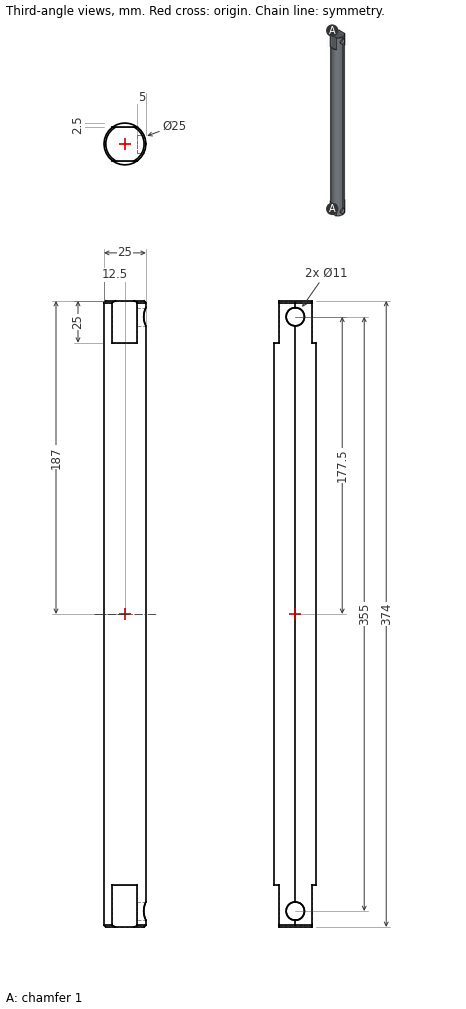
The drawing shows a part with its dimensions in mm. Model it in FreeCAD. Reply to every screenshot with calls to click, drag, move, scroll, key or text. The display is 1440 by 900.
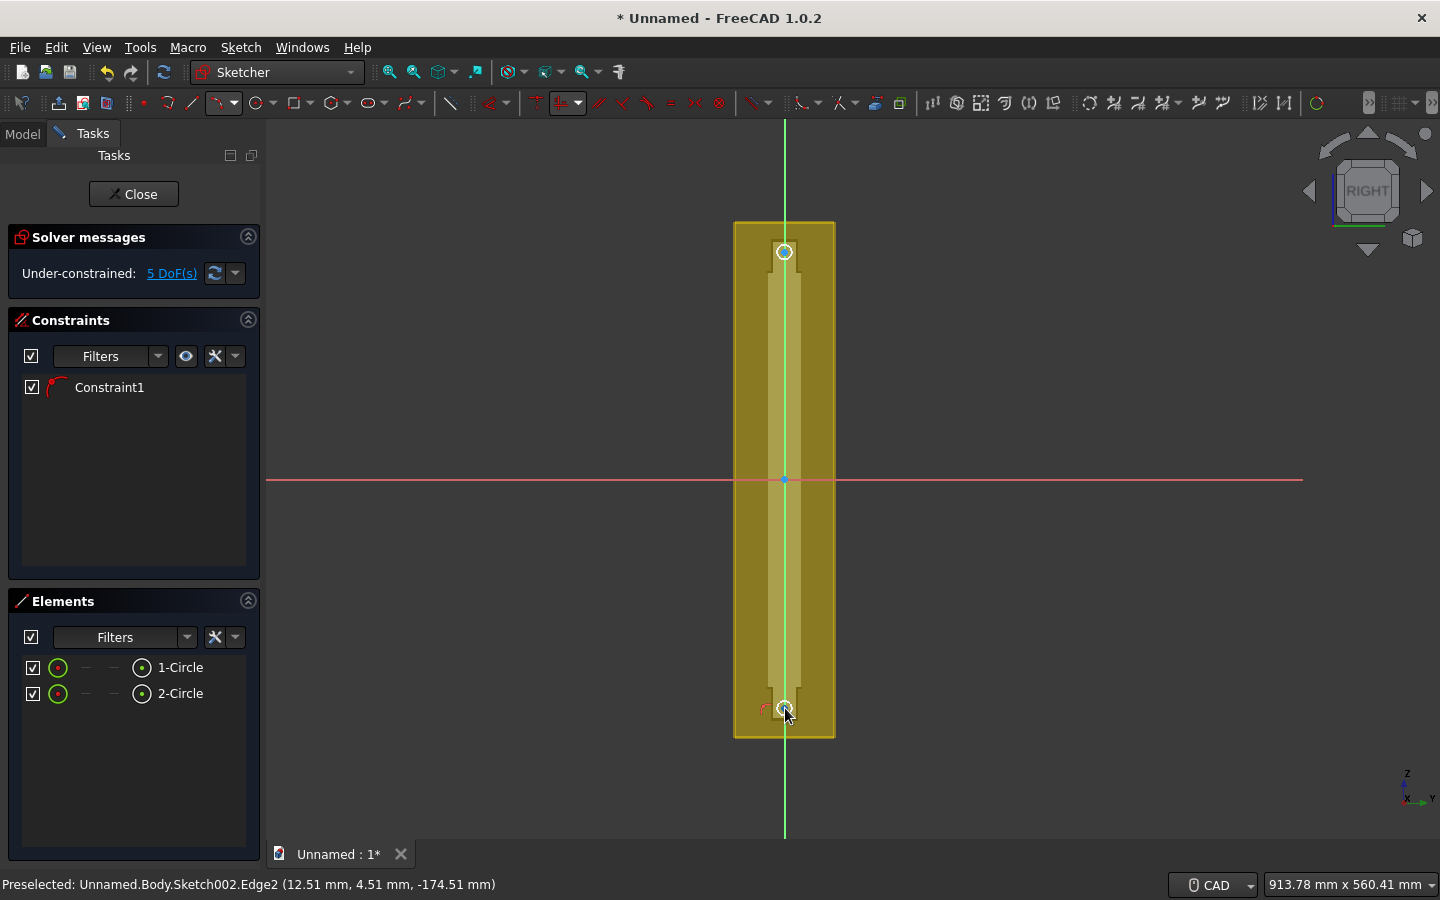
scroll(790, 247, up, 6)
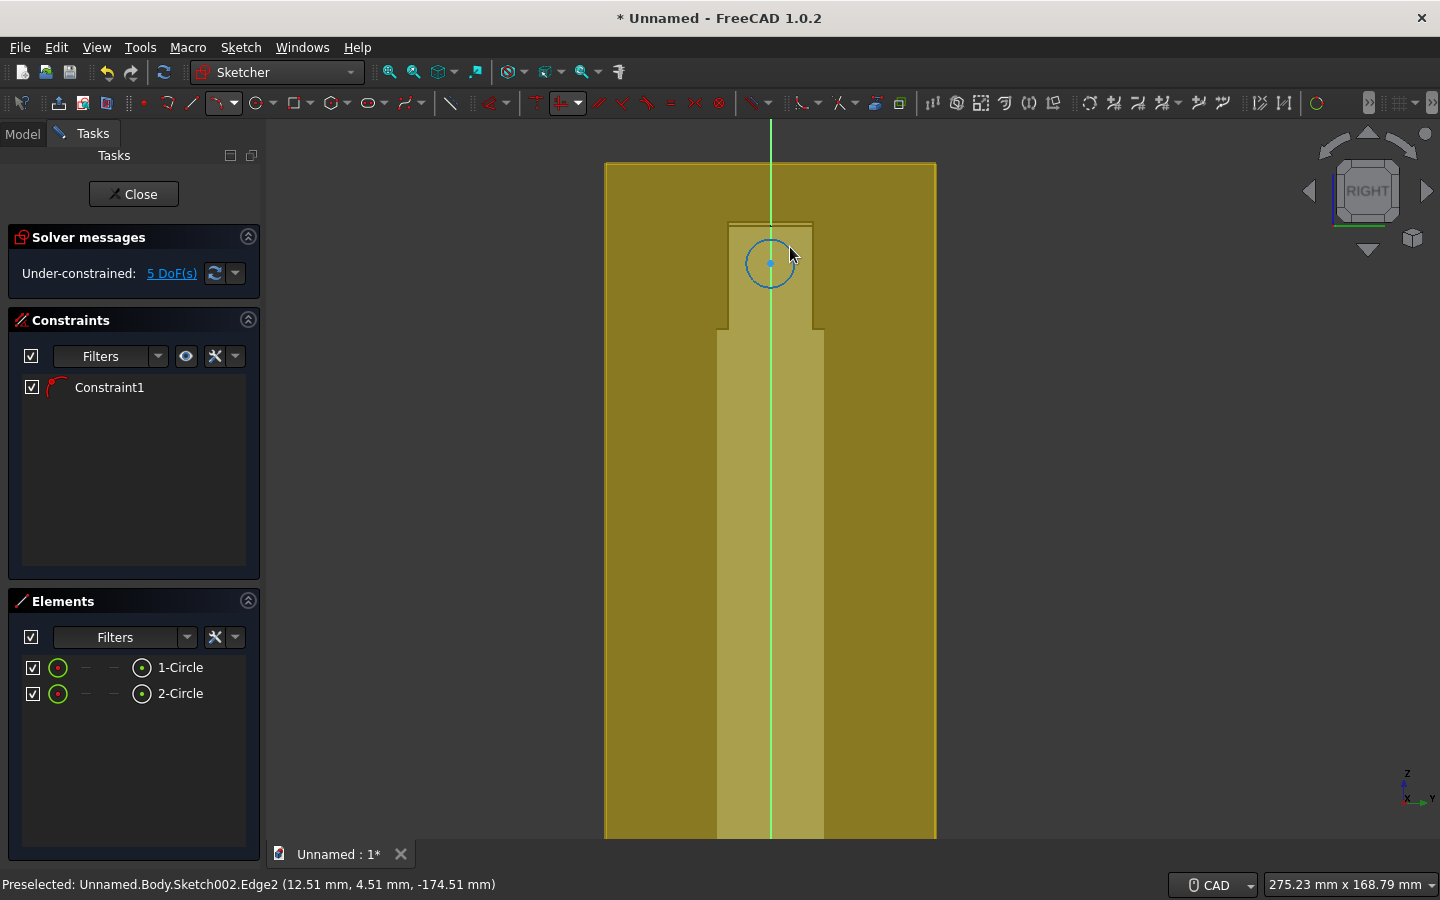
click(787, 247)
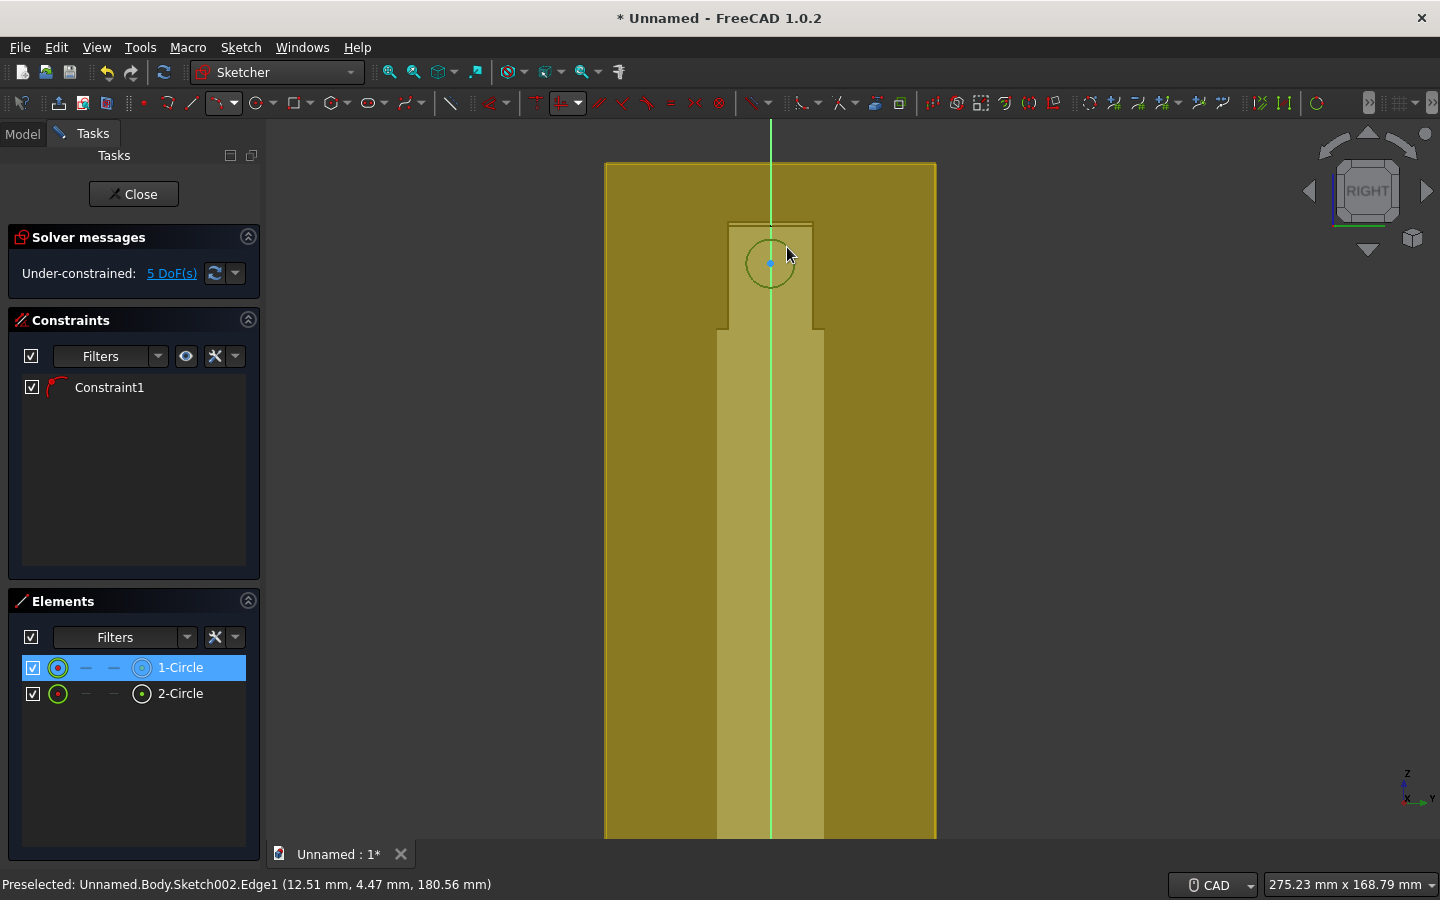
scroll(790, 246, down, 6)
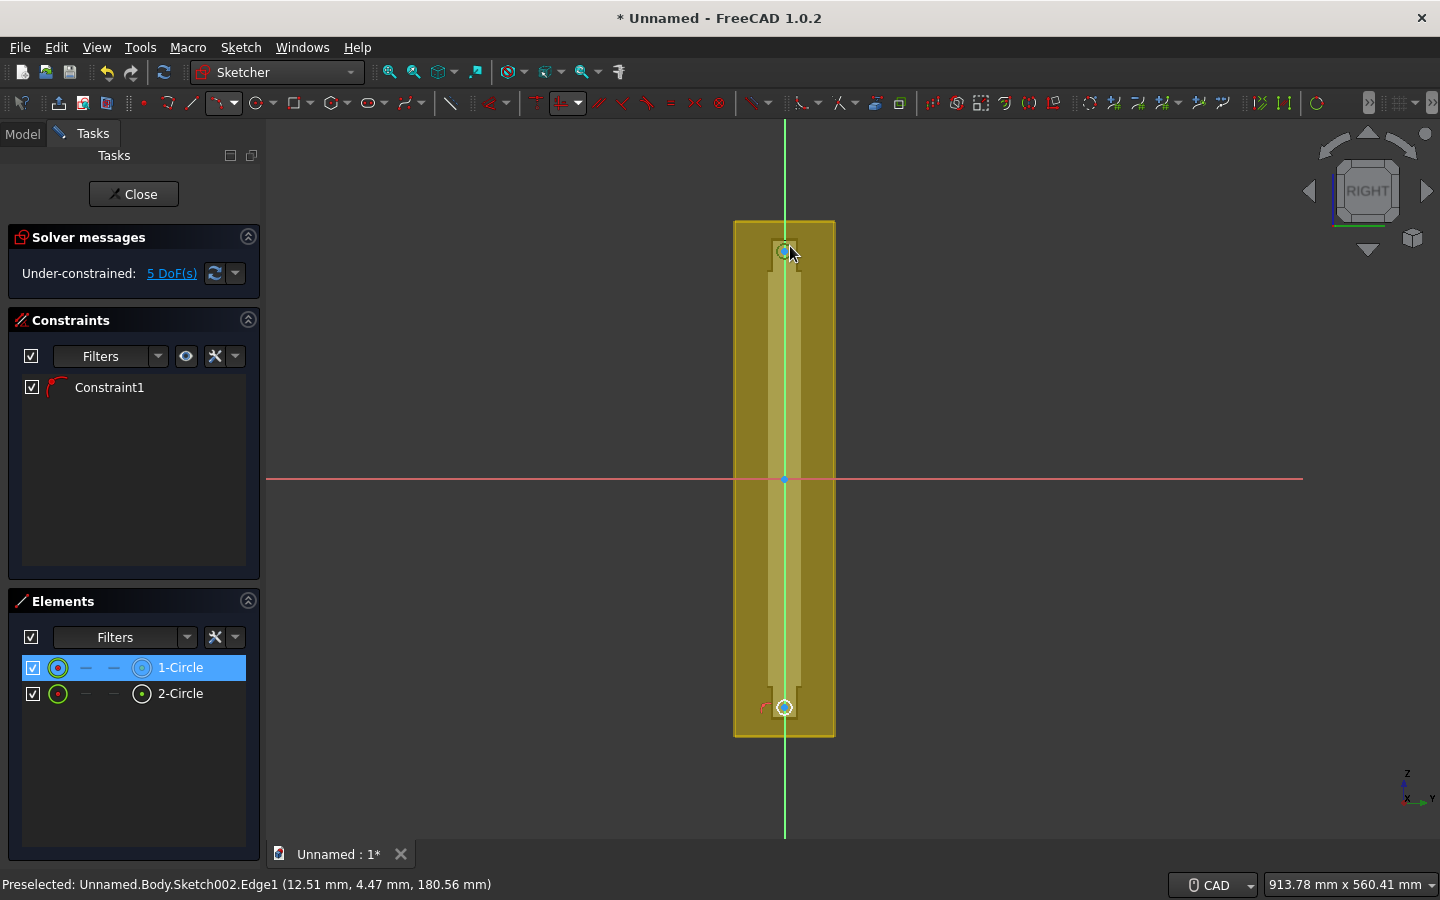
scroll(790, 702, up, 6)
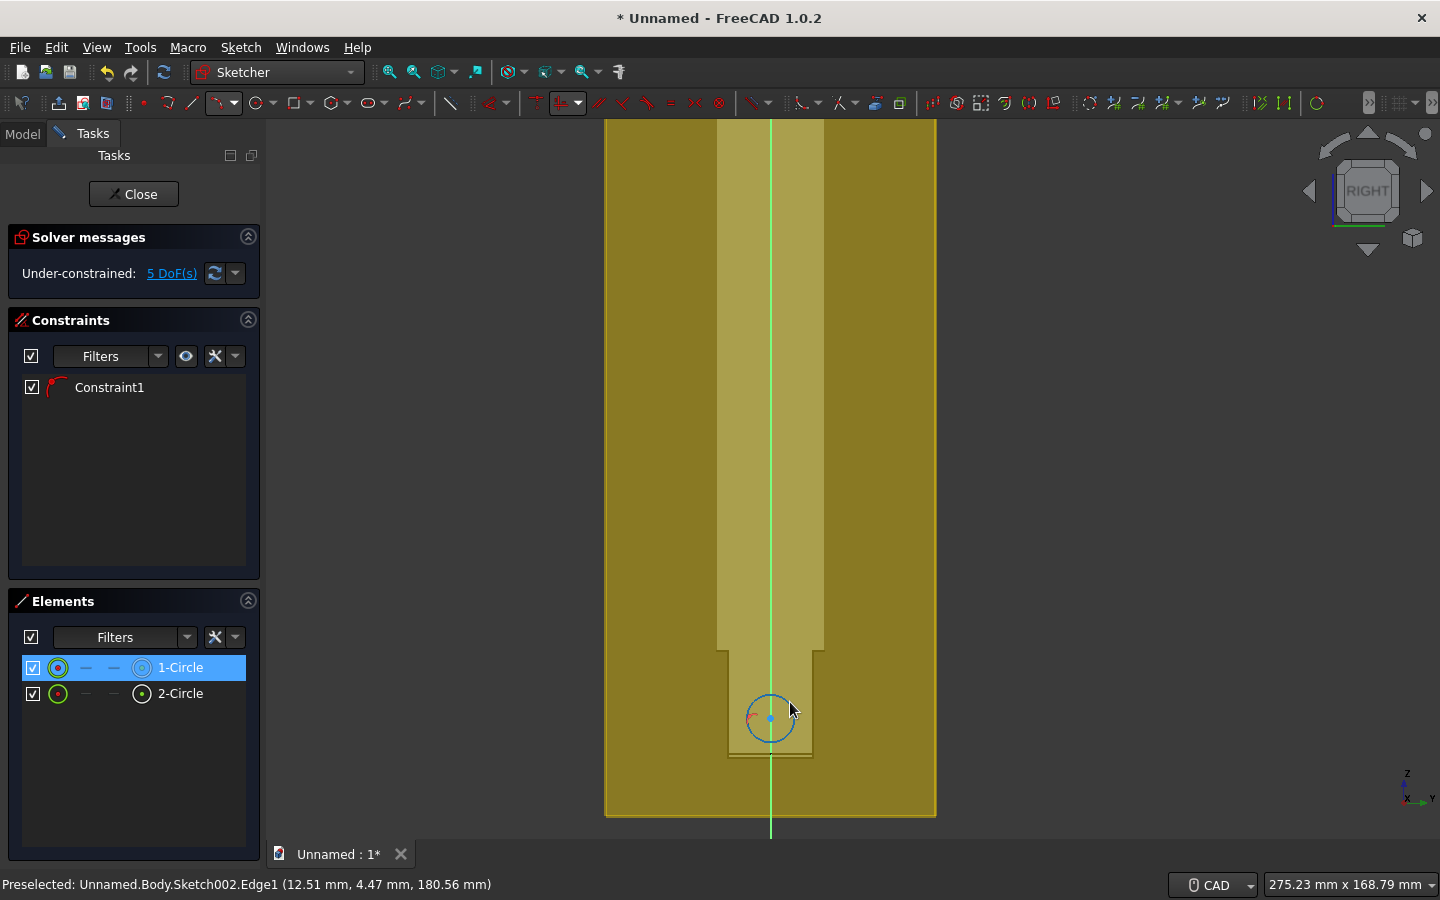
click(788, 702)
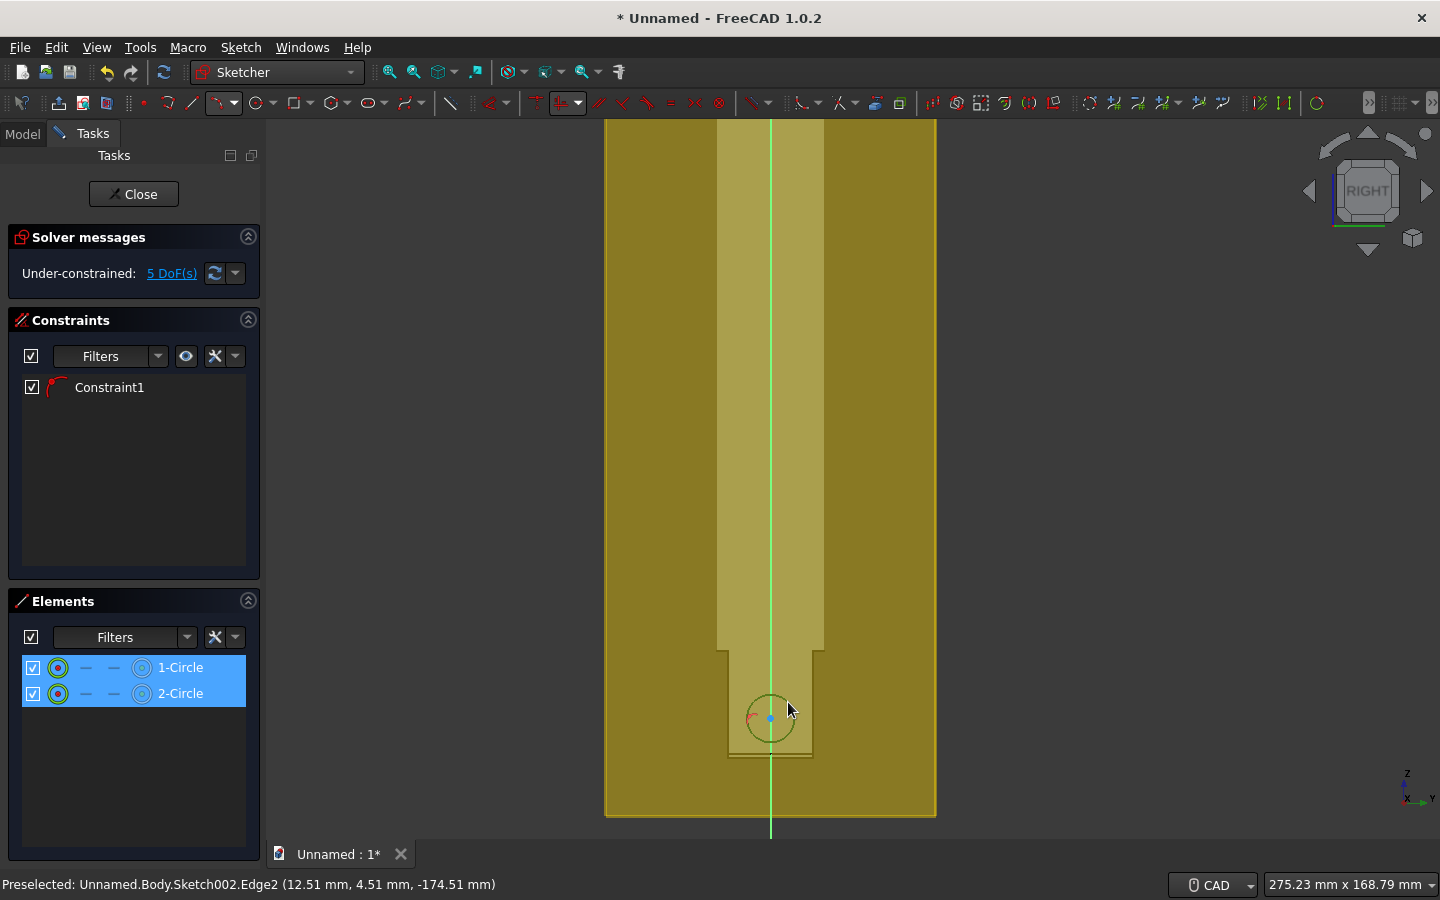
click(672, 104)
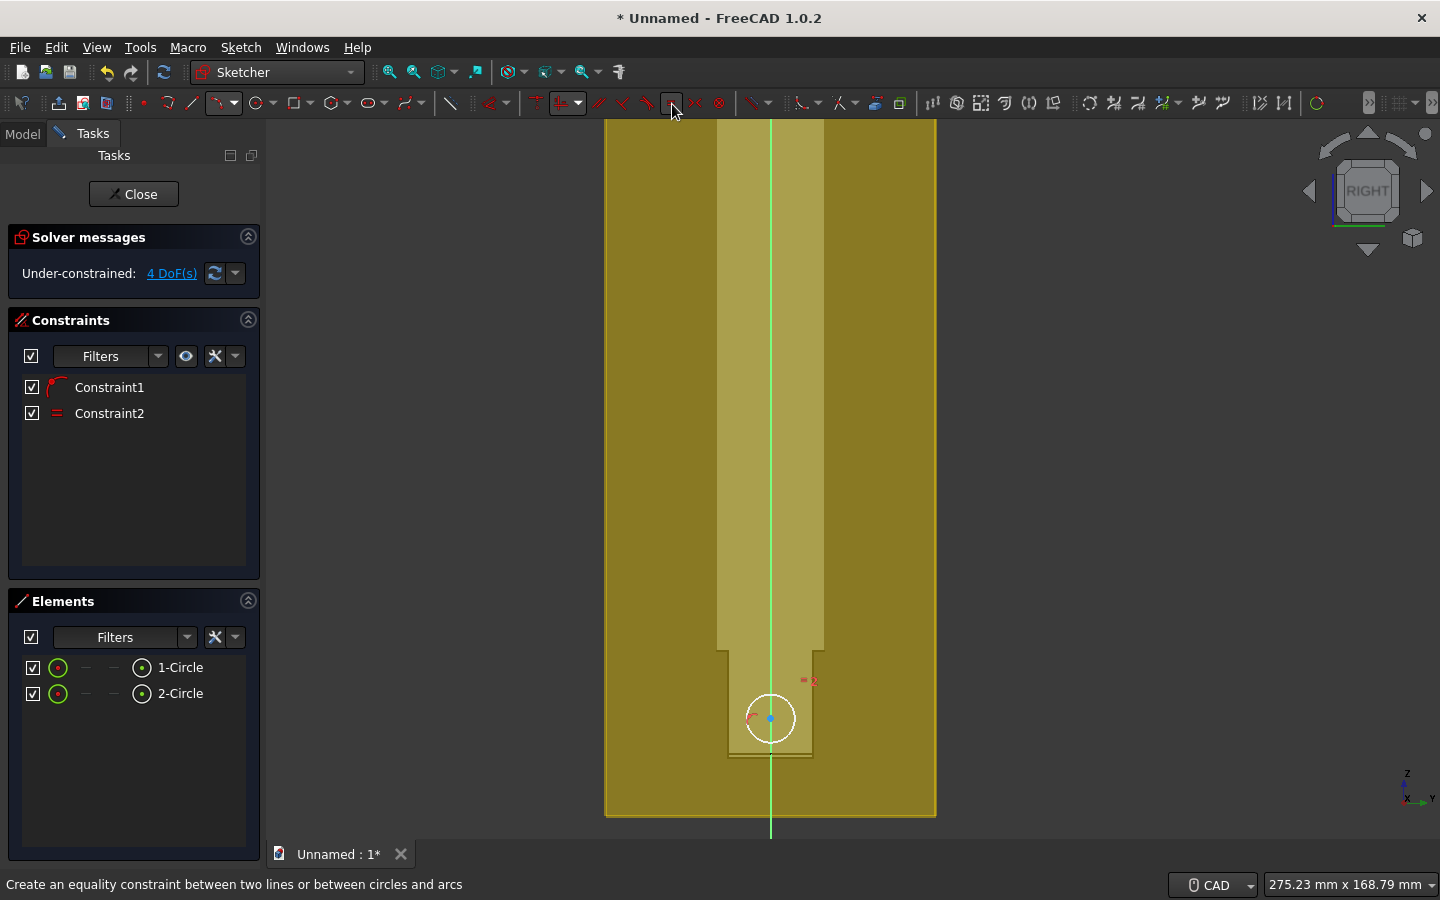
scroll(790, 703, down, 6)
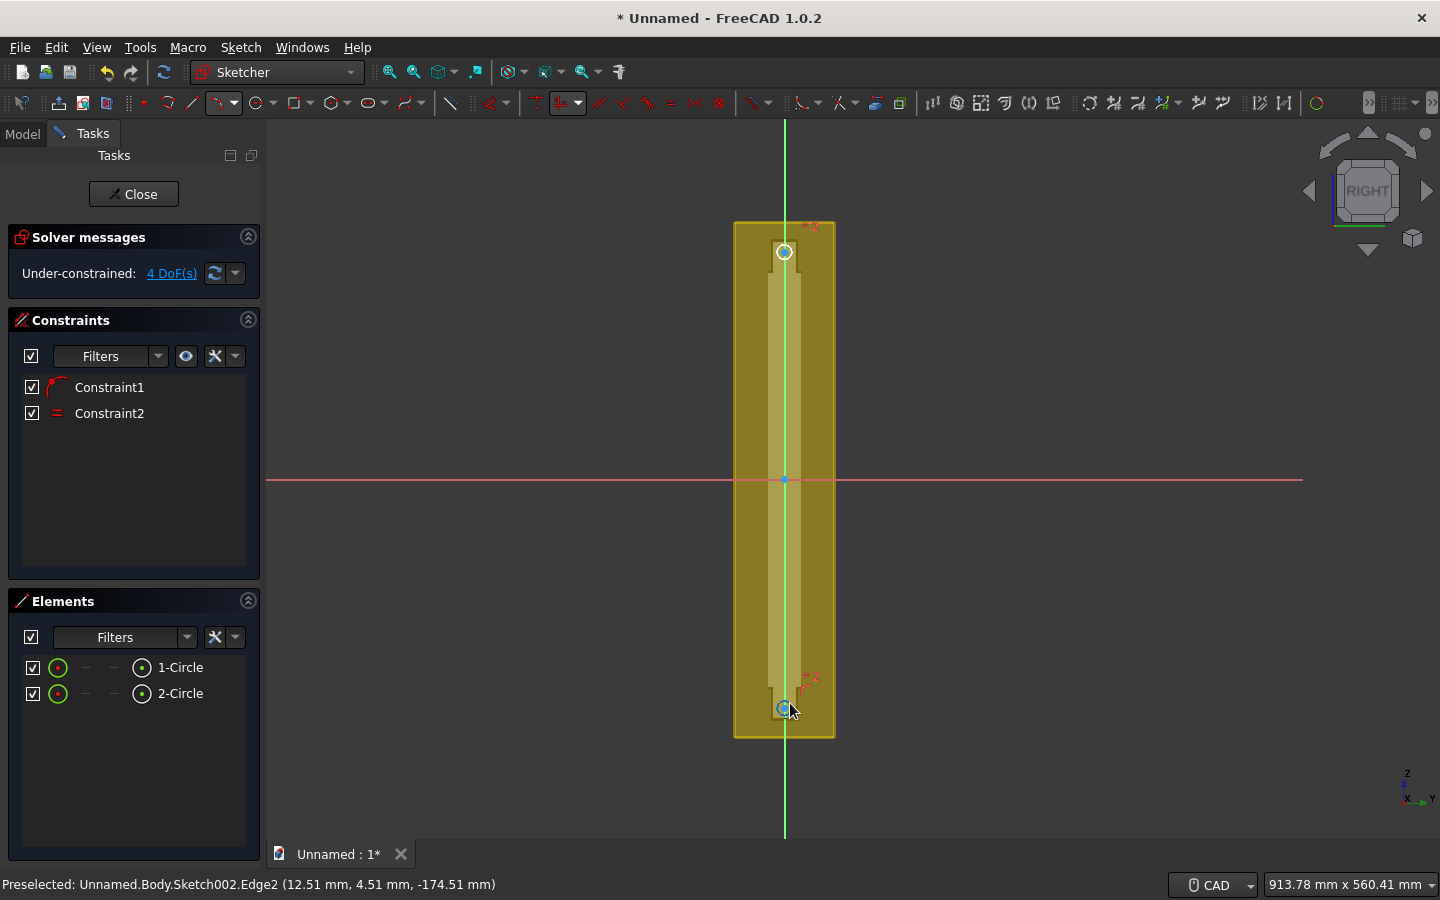
click(784, 252)